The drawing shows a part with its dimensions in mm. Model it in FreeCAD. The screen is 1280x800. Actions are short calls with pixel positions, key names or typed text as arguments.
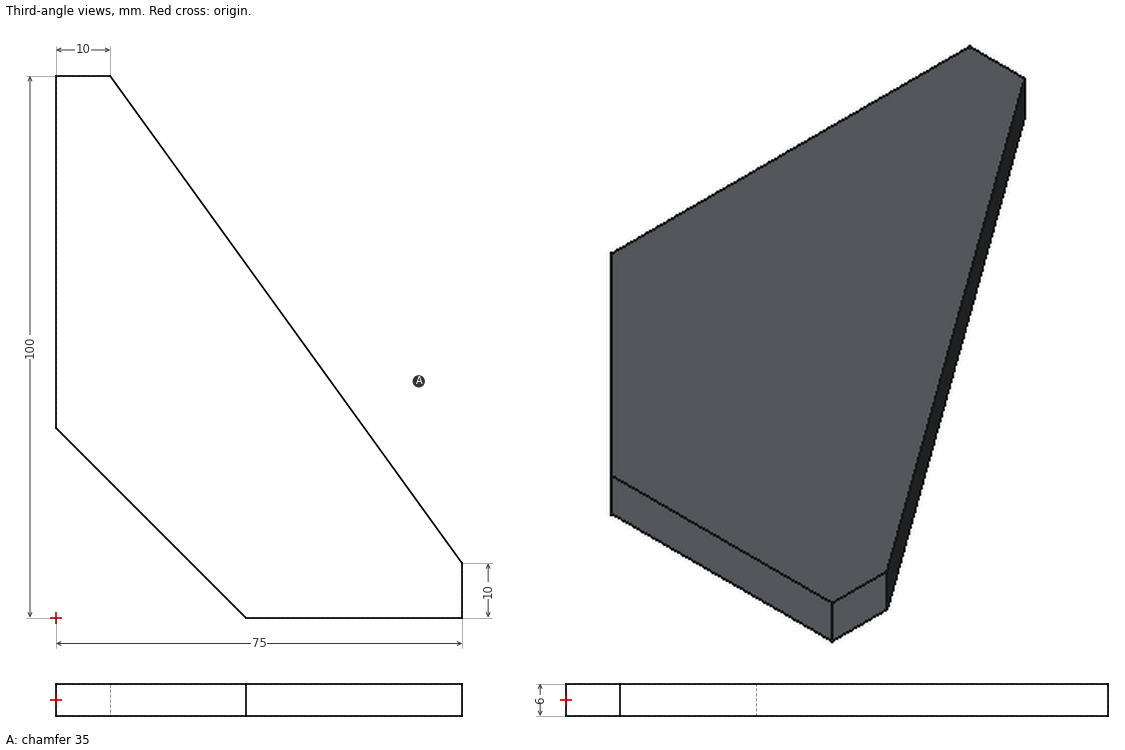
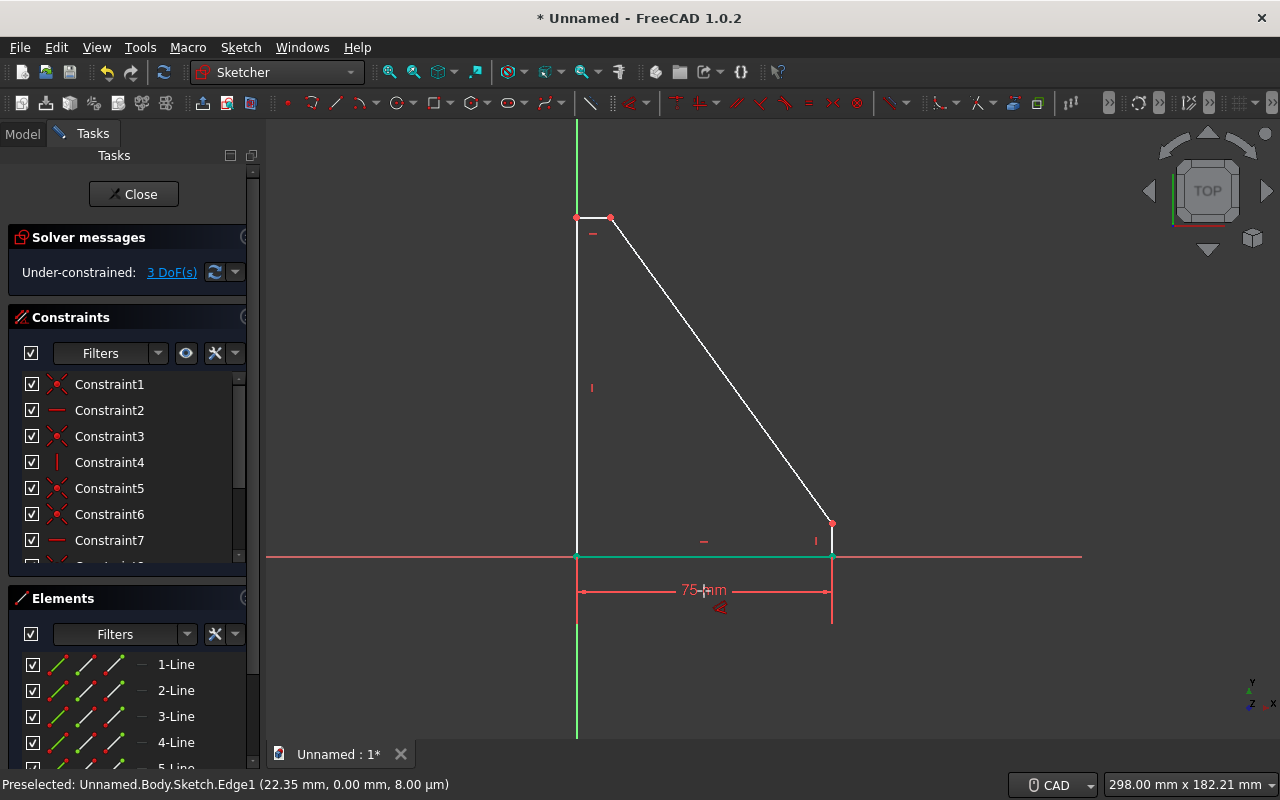
scroll(832, 547, up, 2)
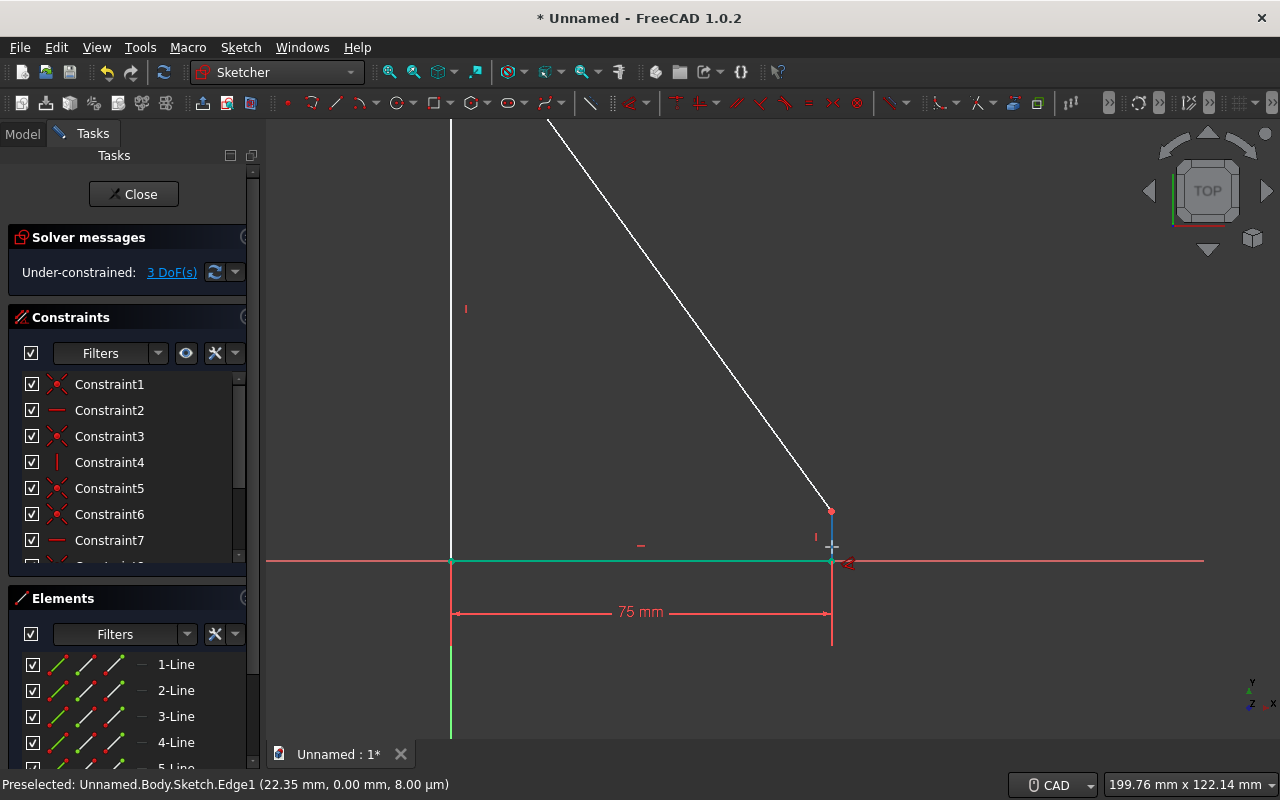
click(832, 546)
click(866, 537)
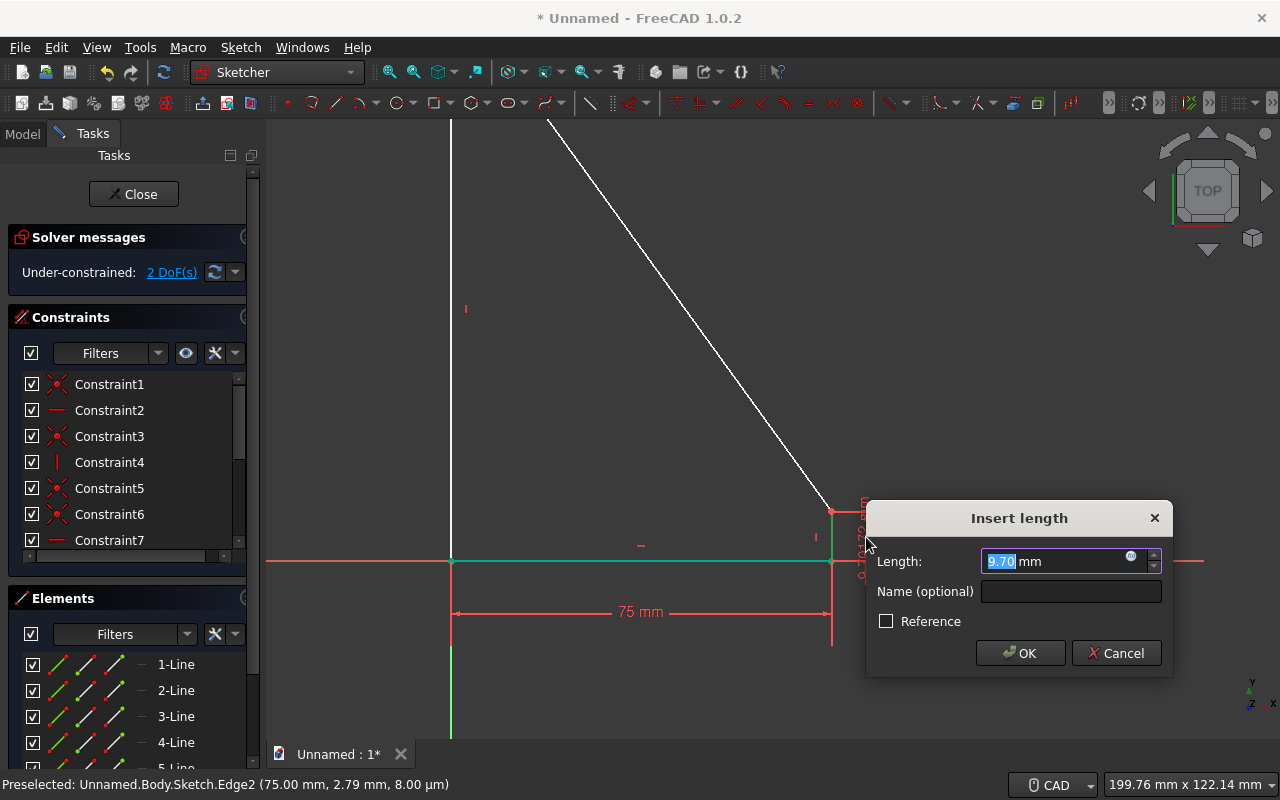
text(10)
key(Return)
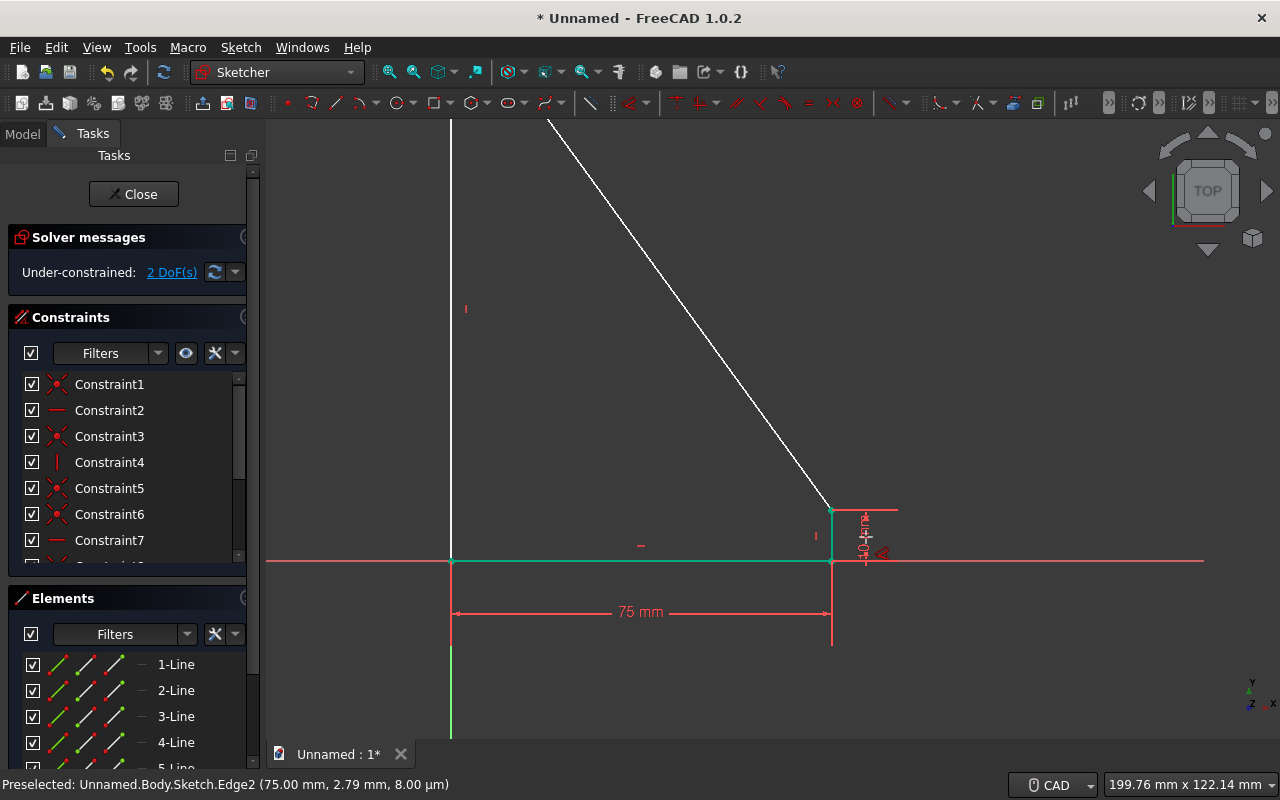
scroll(989, 711, down, 1)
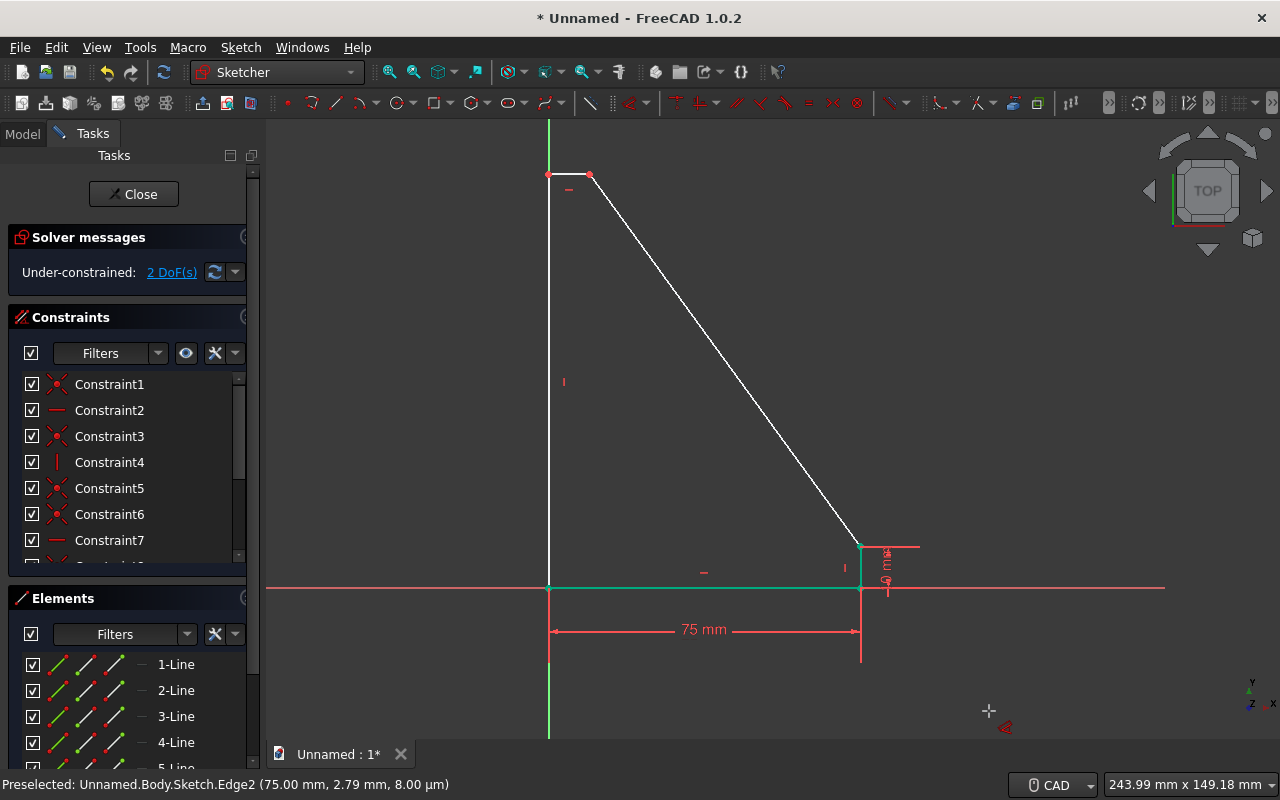
click(578, 174)
click(569, 208)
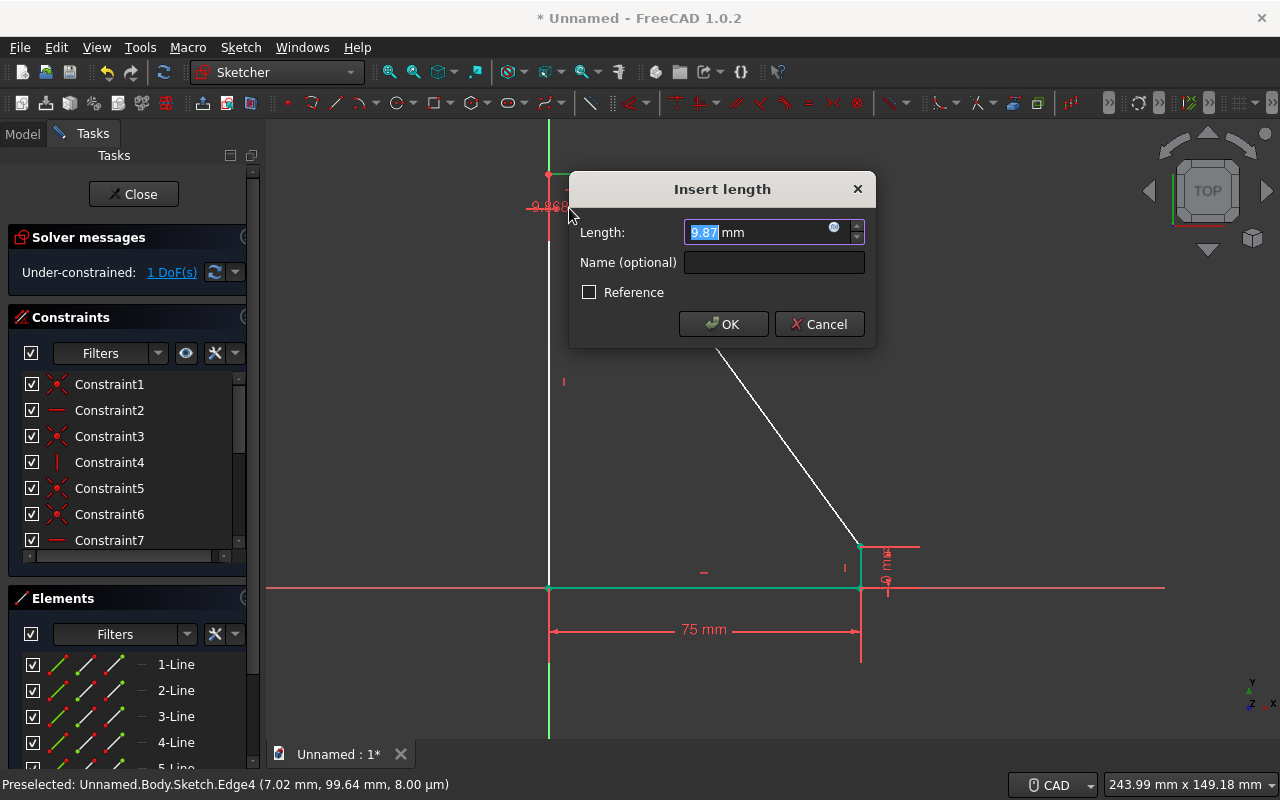
text(10)
key(Return)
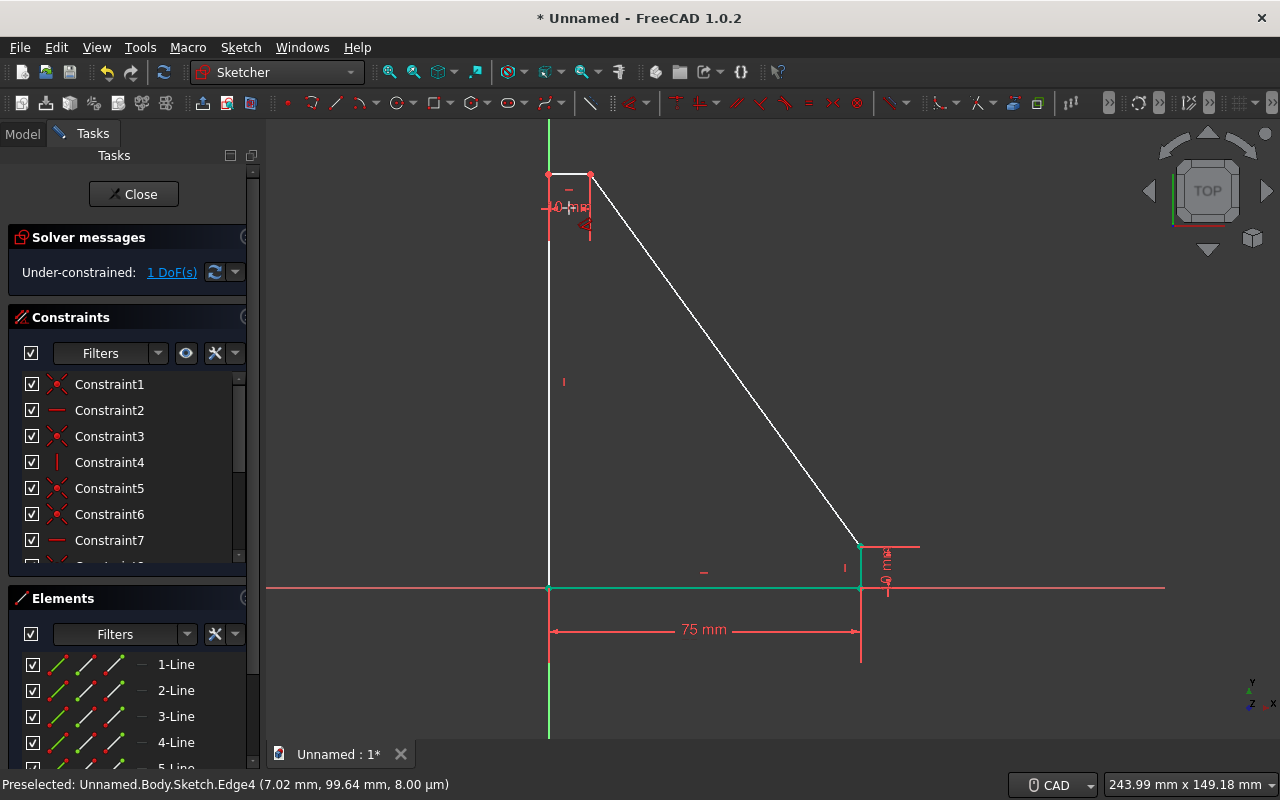
click(549, 299)
click(515, 381)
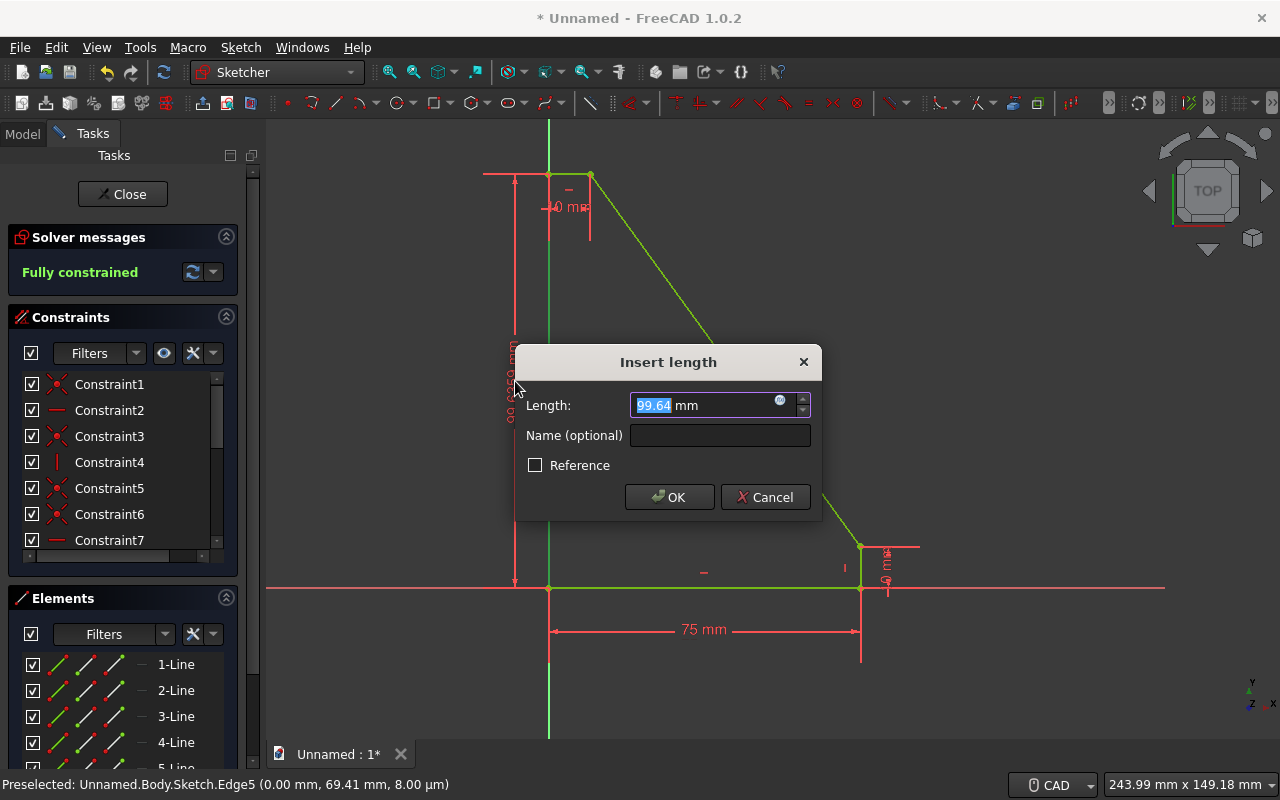
text(100)
key(Return)
key(Escape)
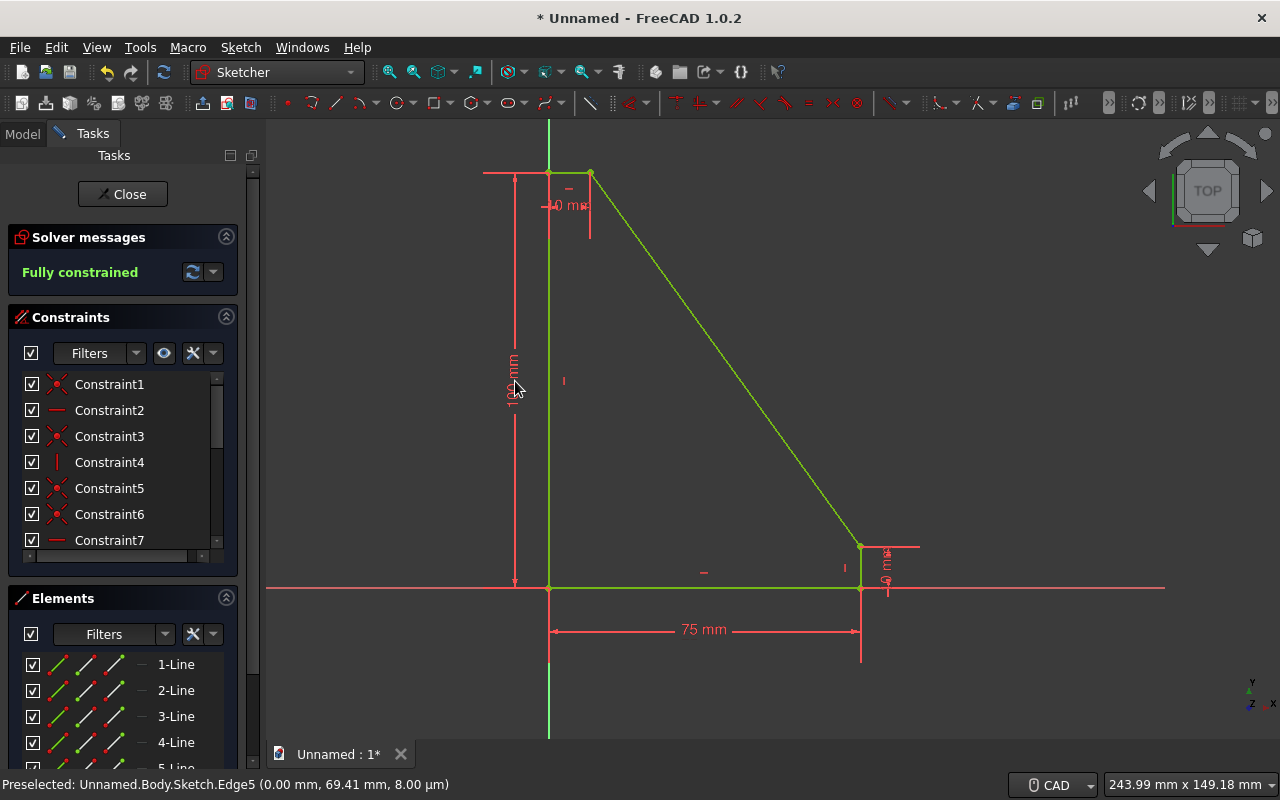
click(123, 194)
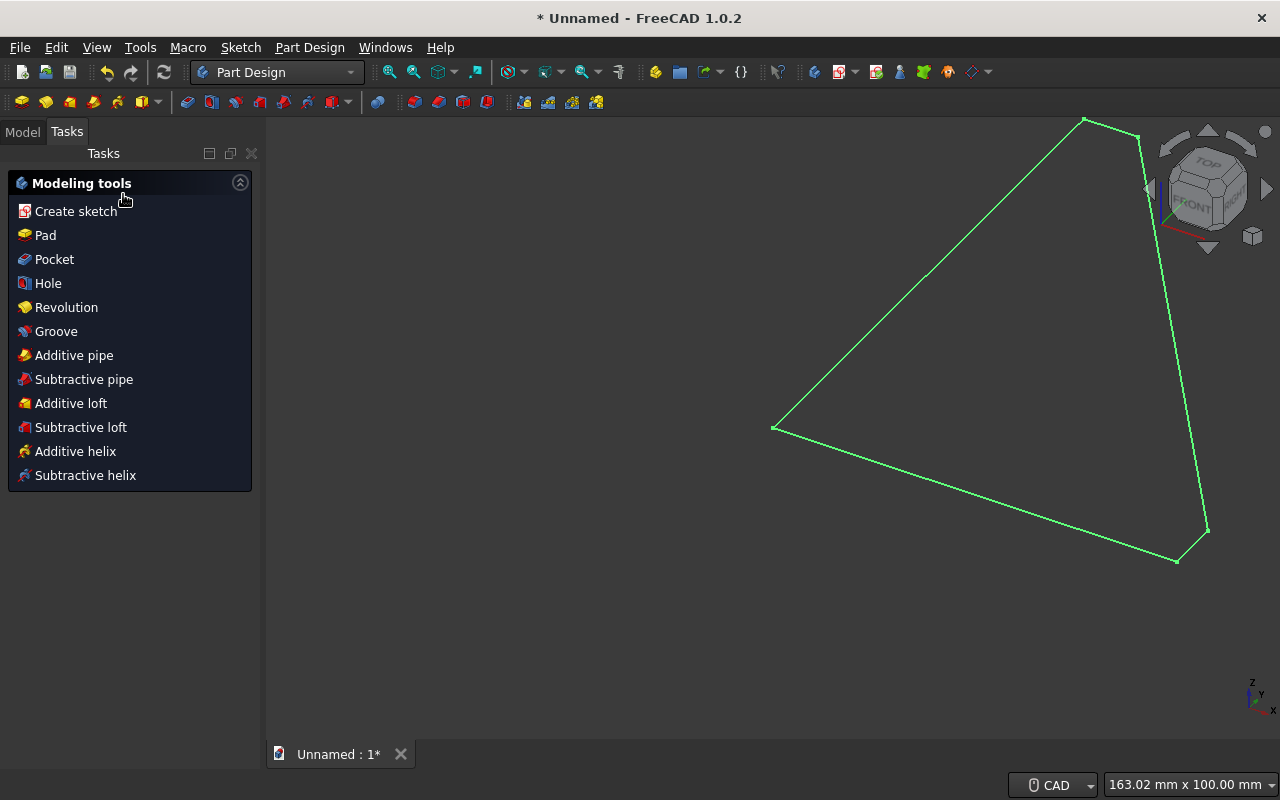
click(22, 102)